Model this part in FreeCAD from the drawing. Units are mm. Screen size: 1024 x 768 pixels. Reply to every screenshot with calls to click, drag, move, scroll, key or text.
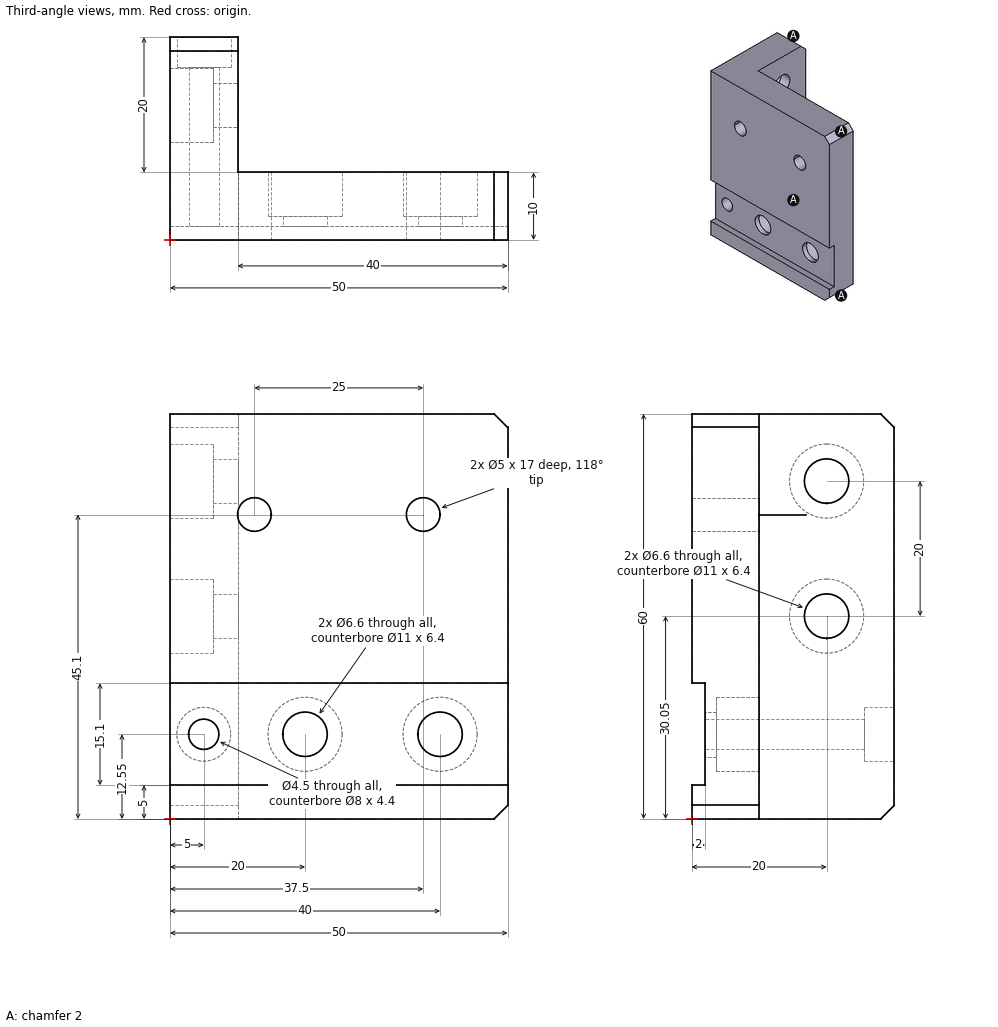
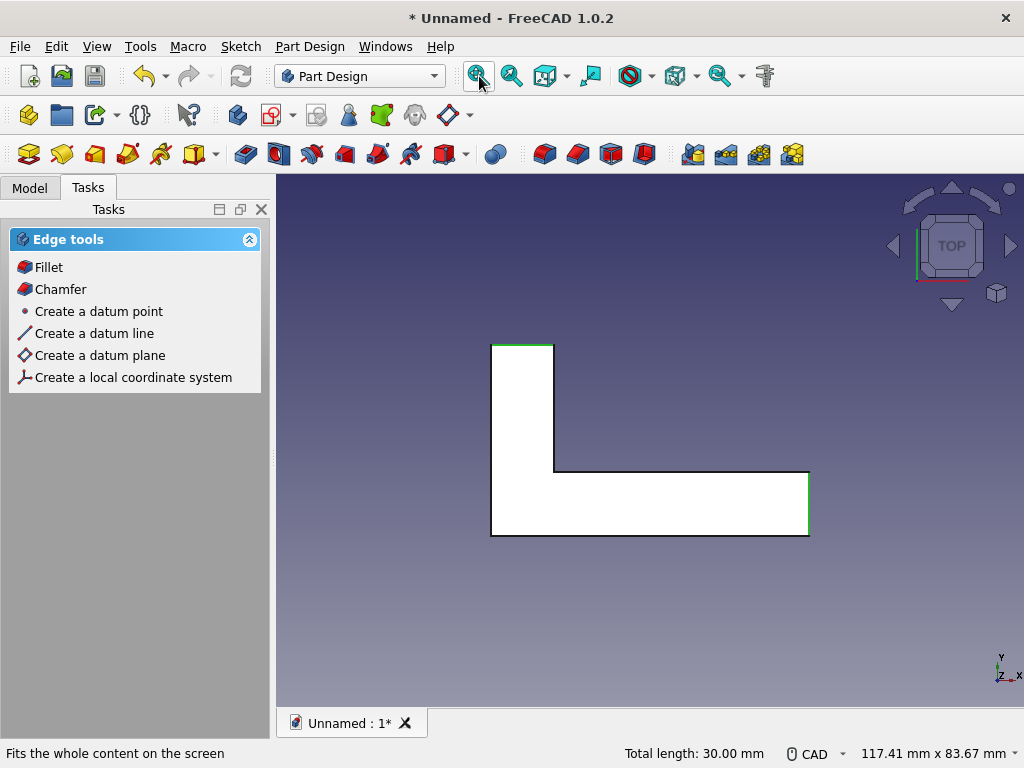
key(1)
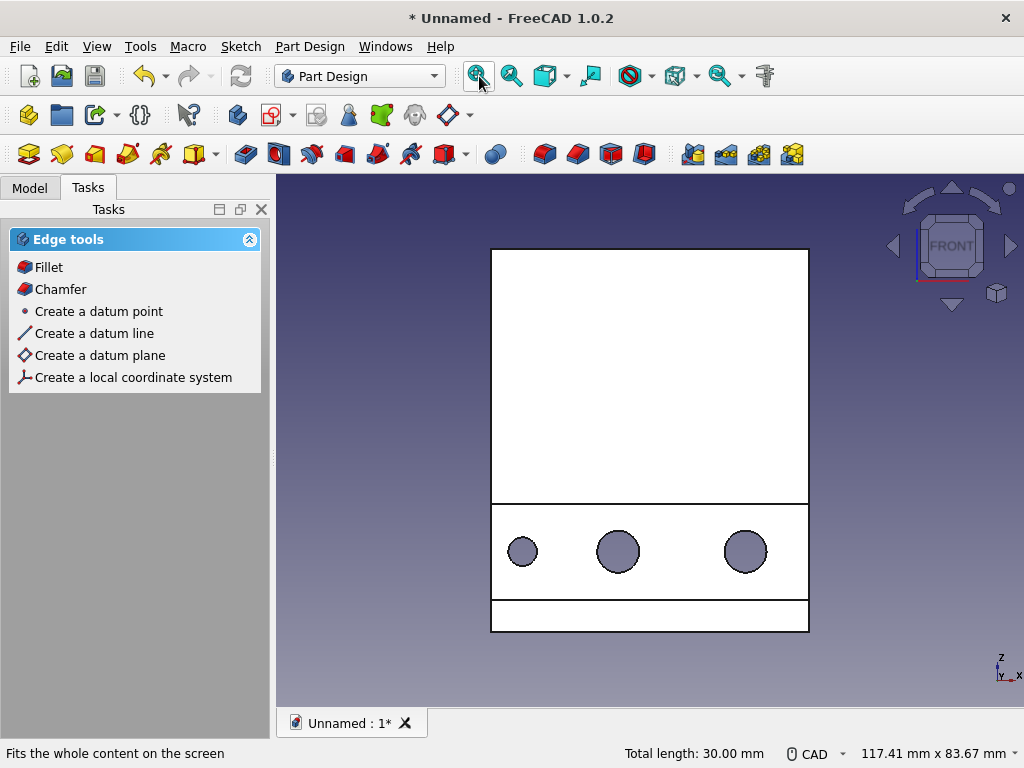
key(3)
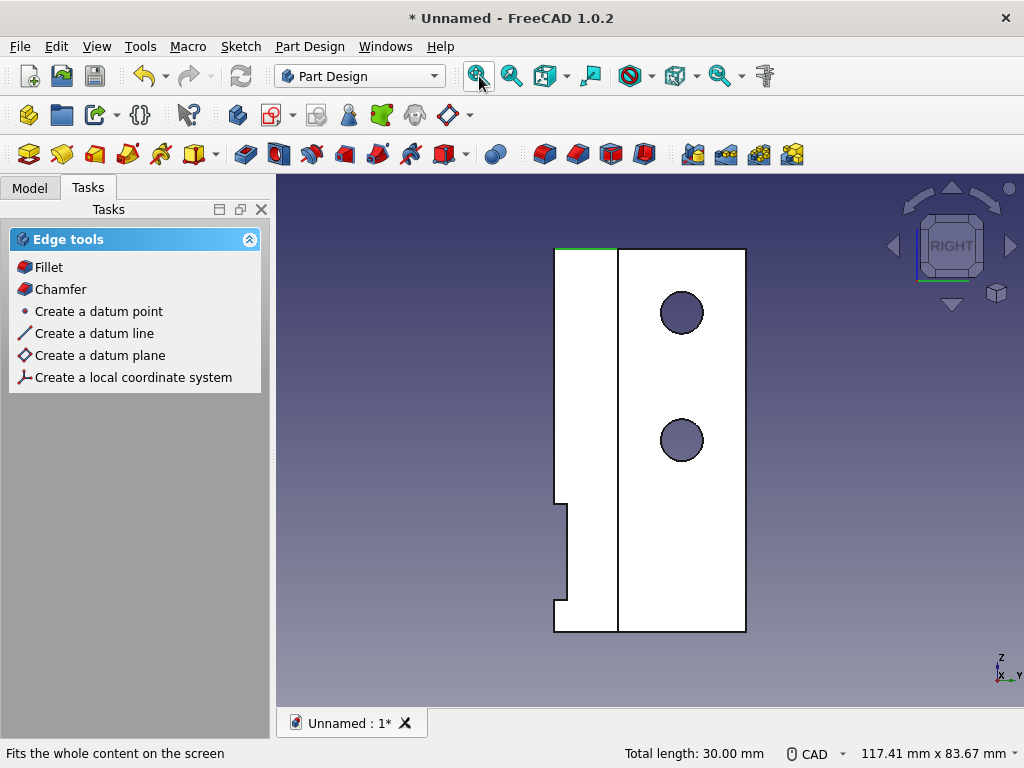
click(586, 631, ctrl)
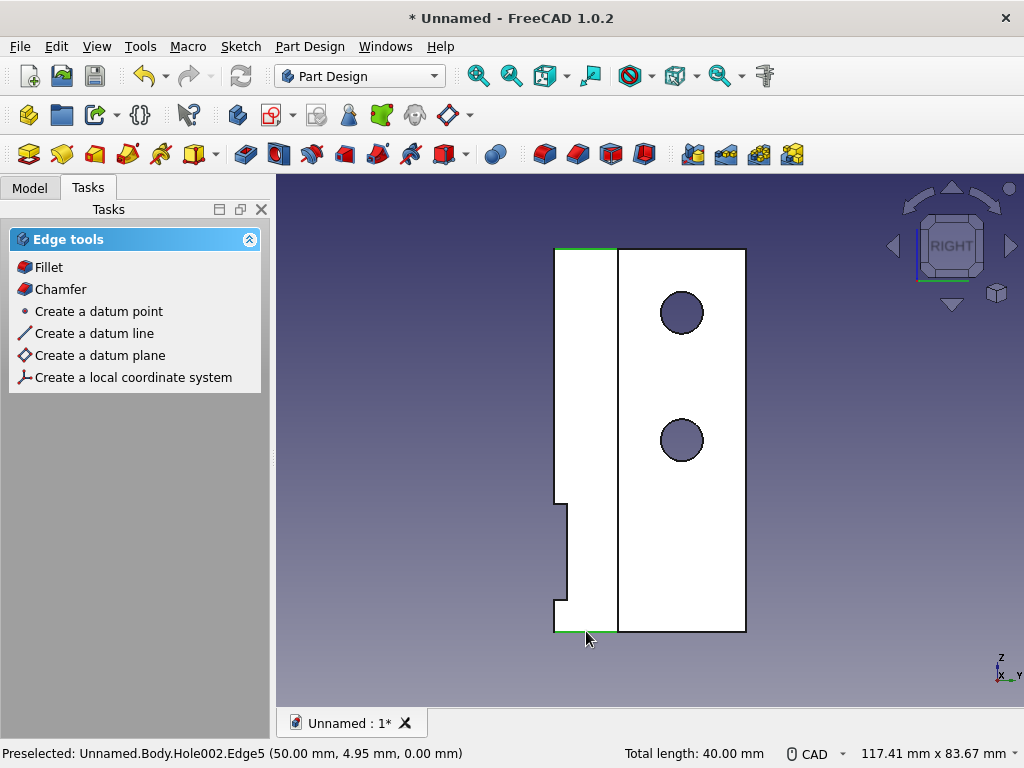
click(578, 154)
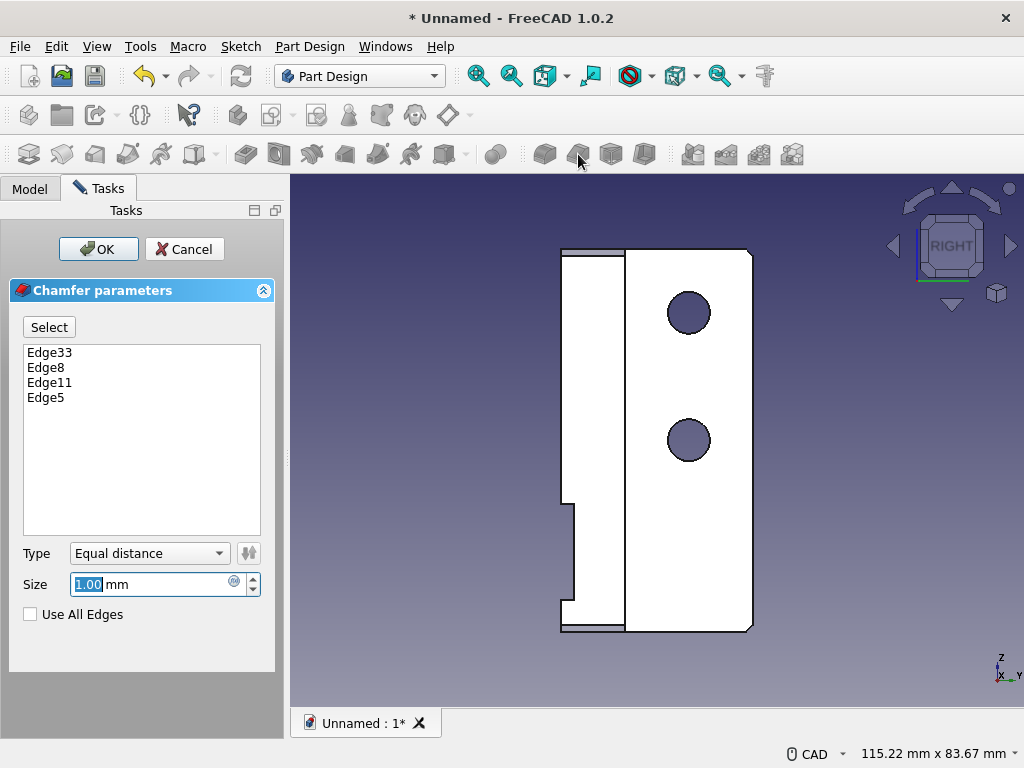
text(2)
key(Tab)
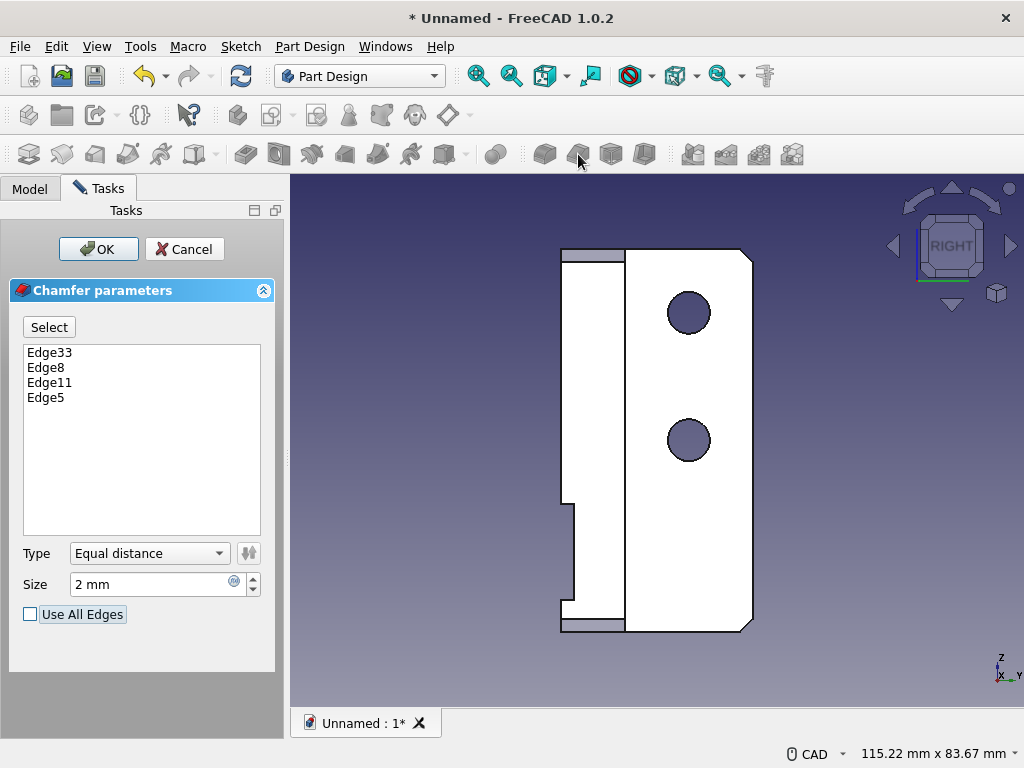
click(99, 249)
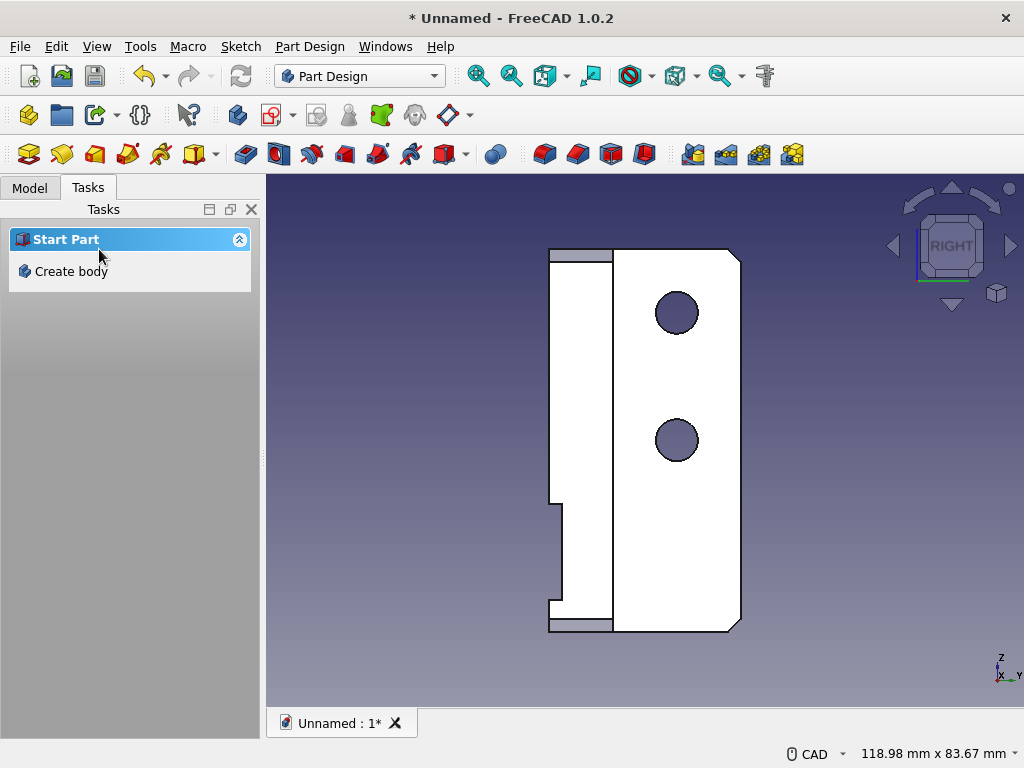
key(0)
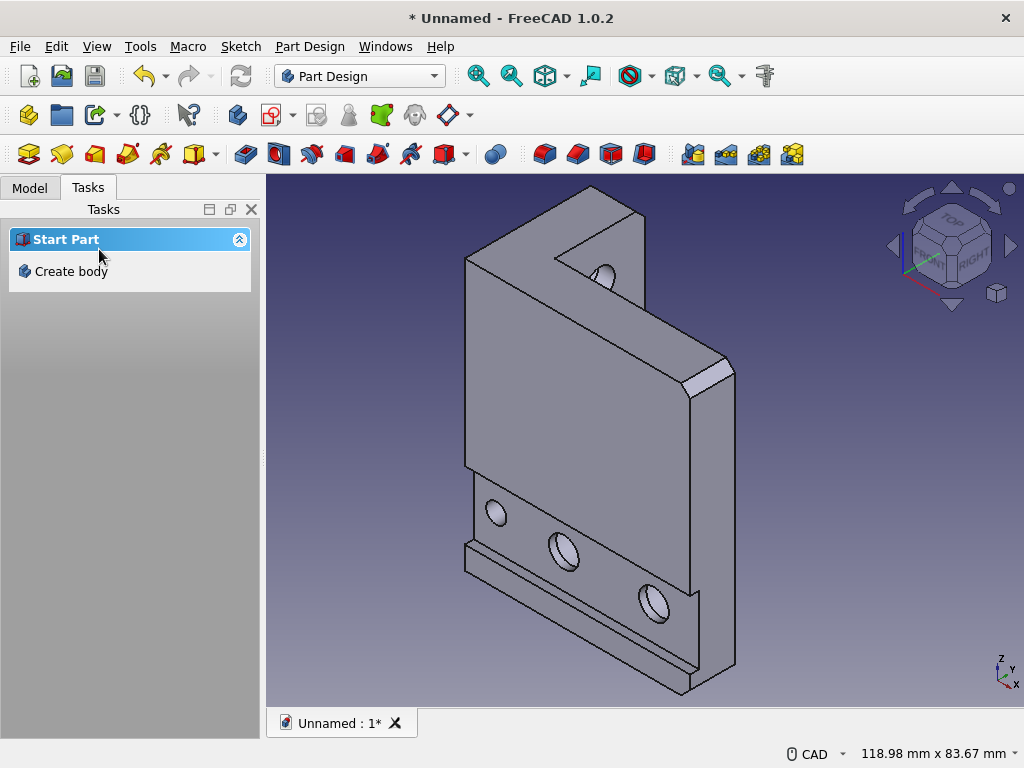
click(577, 426)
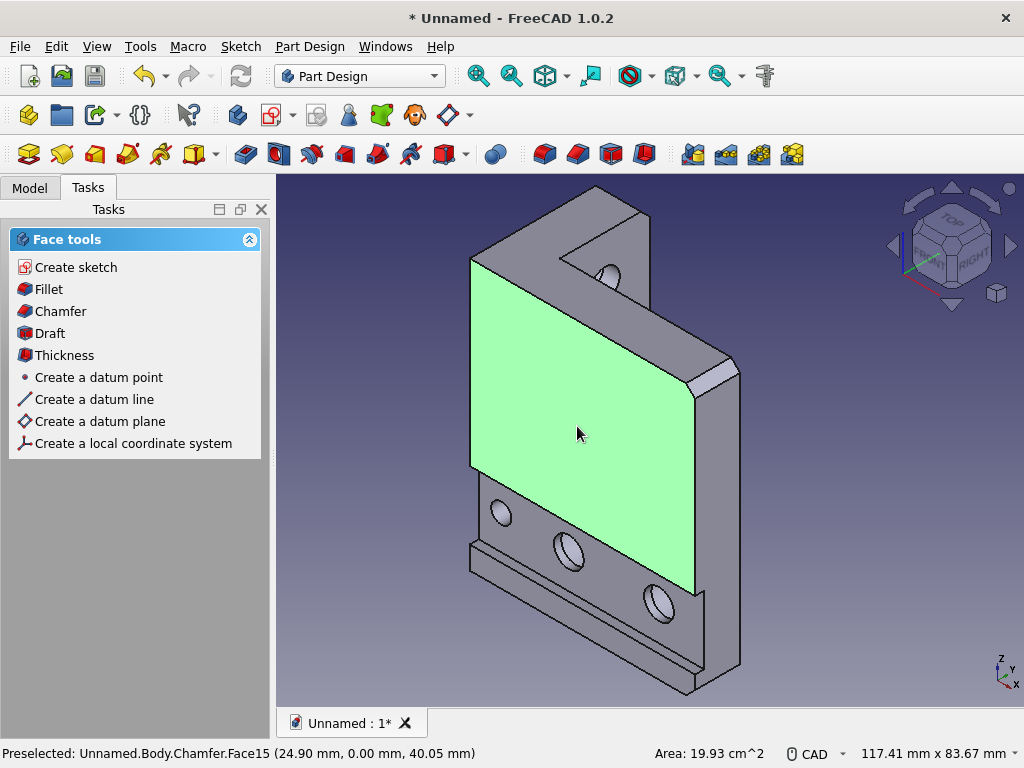
click(270, 116)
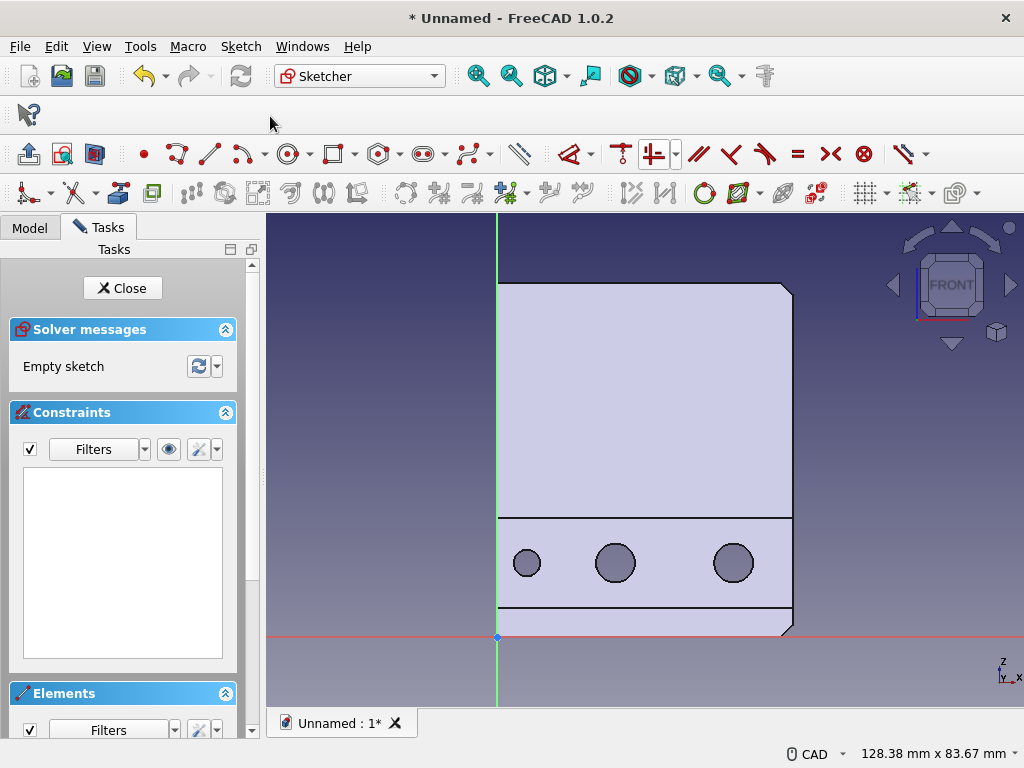
click(288, 154)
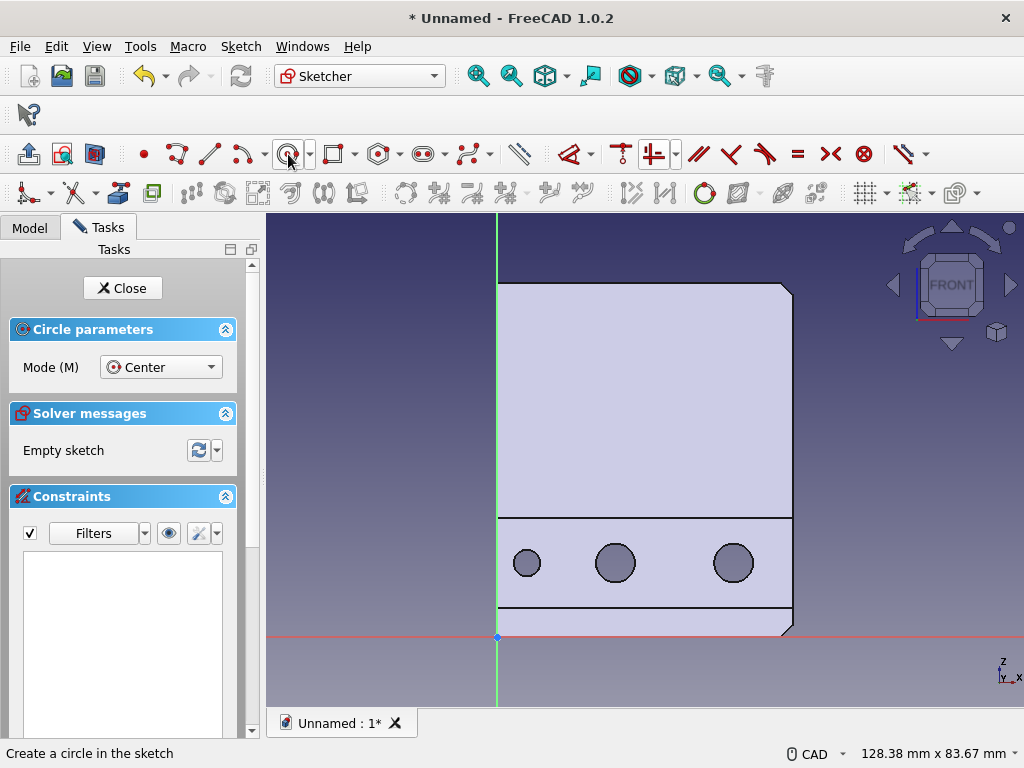
scroll(719, 371, up, 3)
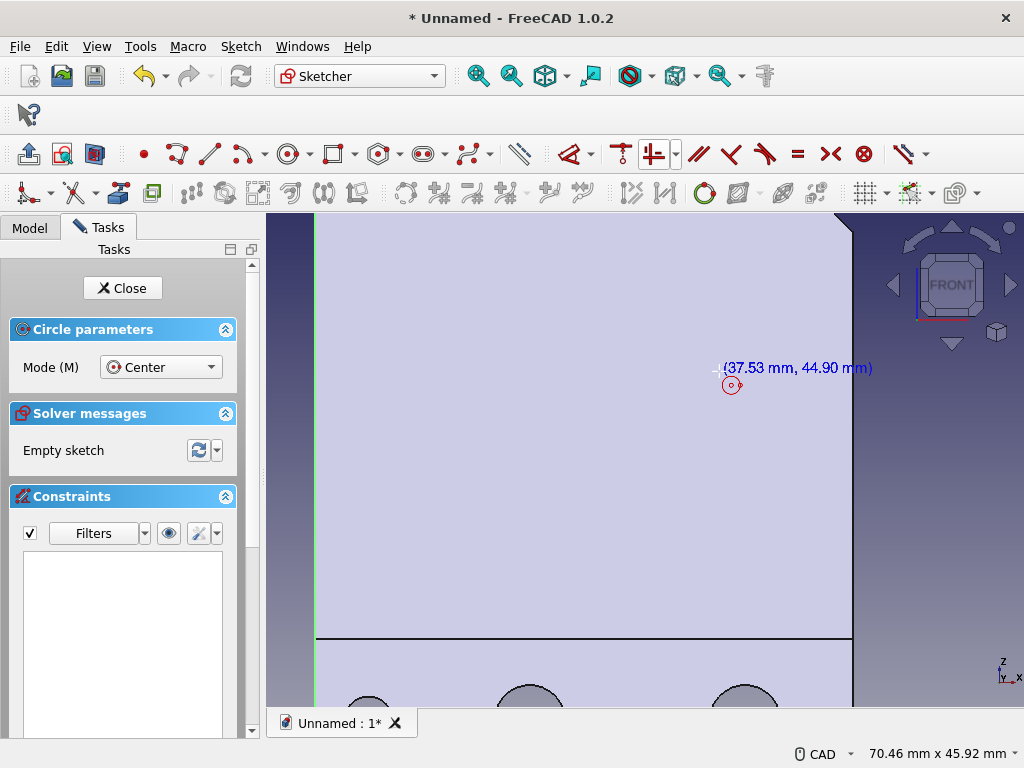
click(718, 370)
click(737, 351)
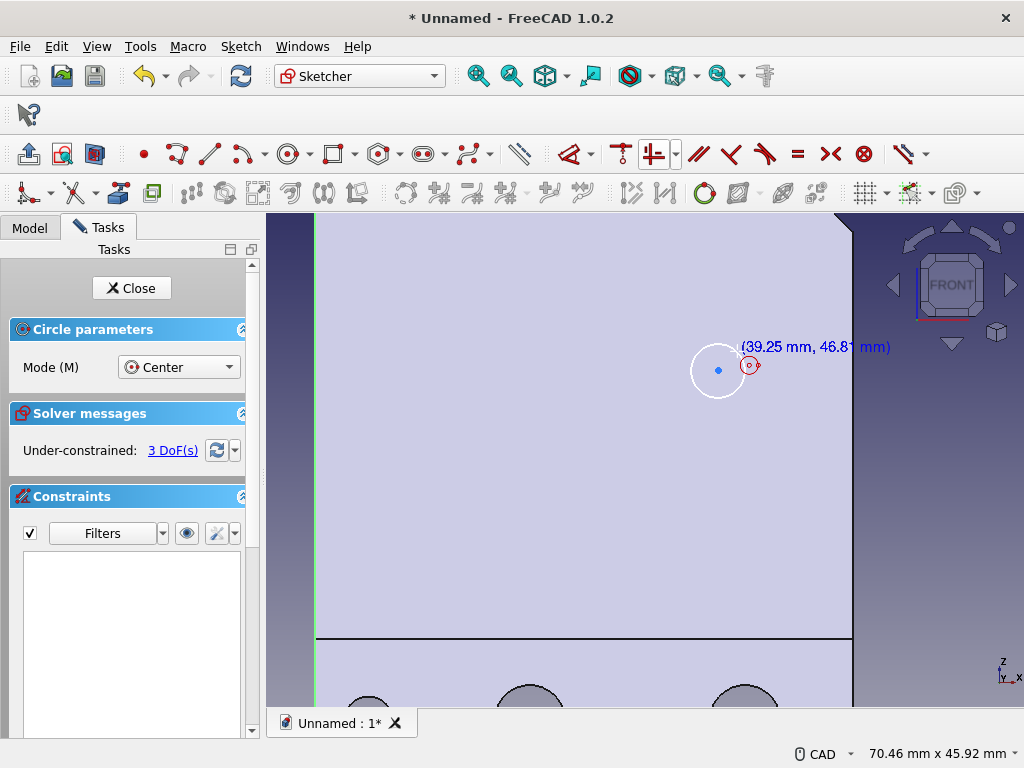
click(449, 370)
click(468, 351)
key(Escape)